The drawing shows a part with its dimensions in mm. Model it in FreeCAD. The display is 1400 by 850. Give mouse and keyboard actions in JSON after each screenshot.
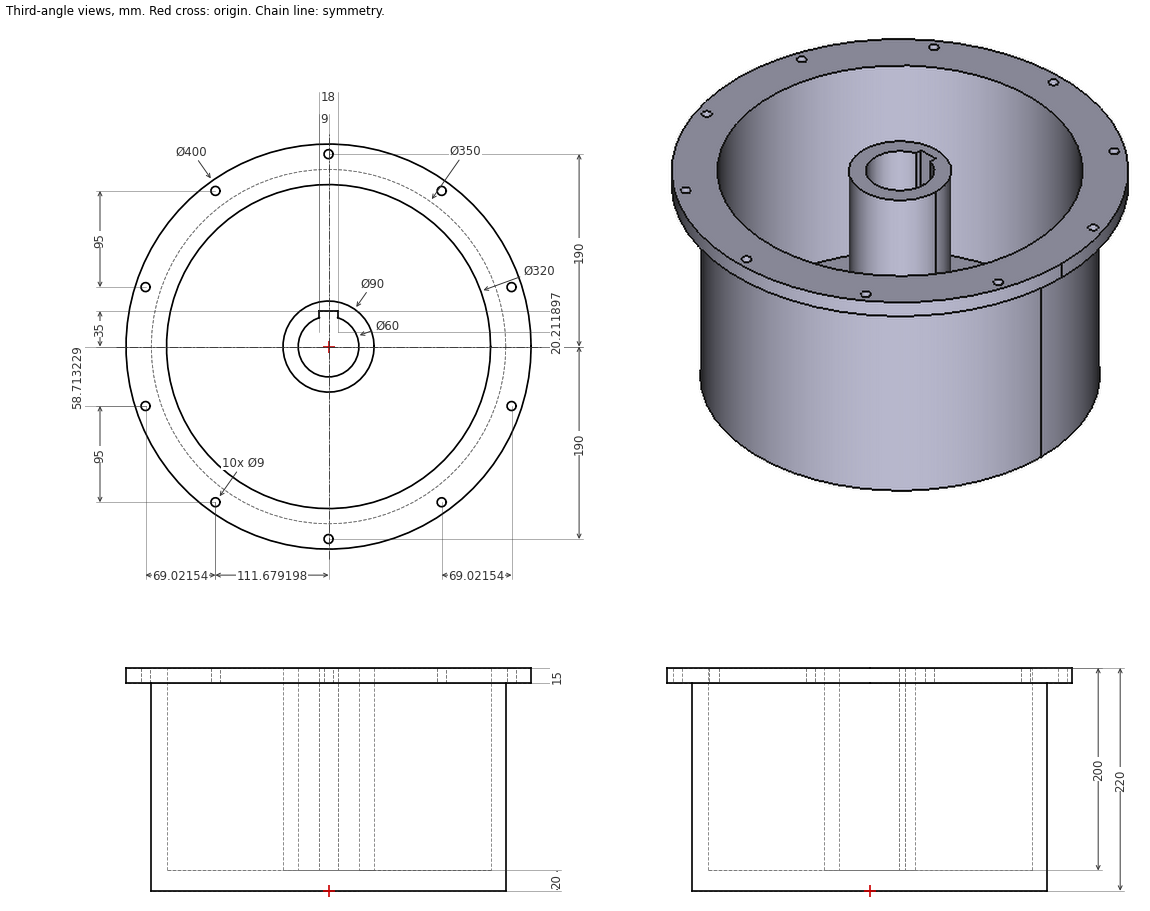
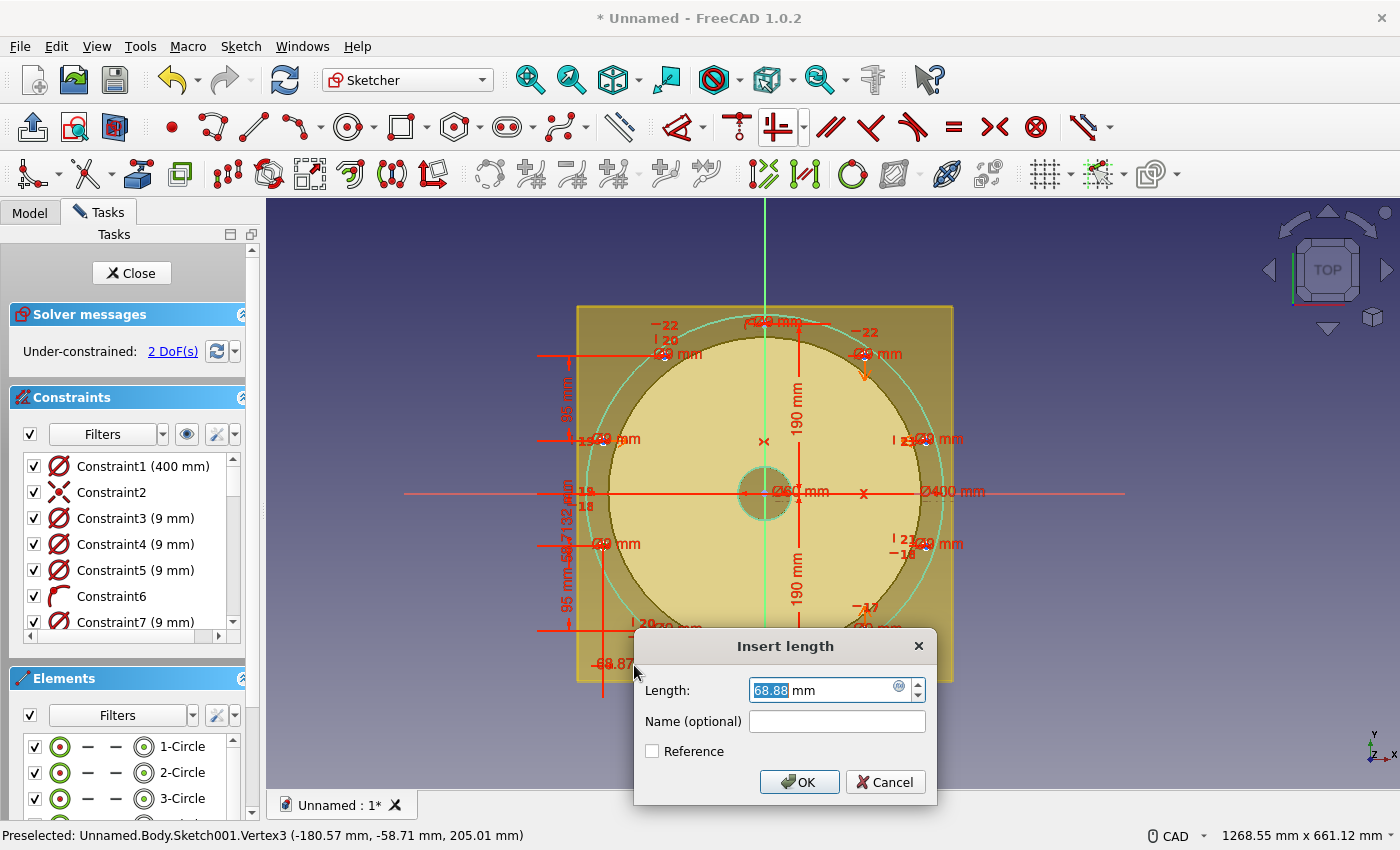
{"action": "type", "text": "69.02154"}
{"action": "key", "text": "Return"}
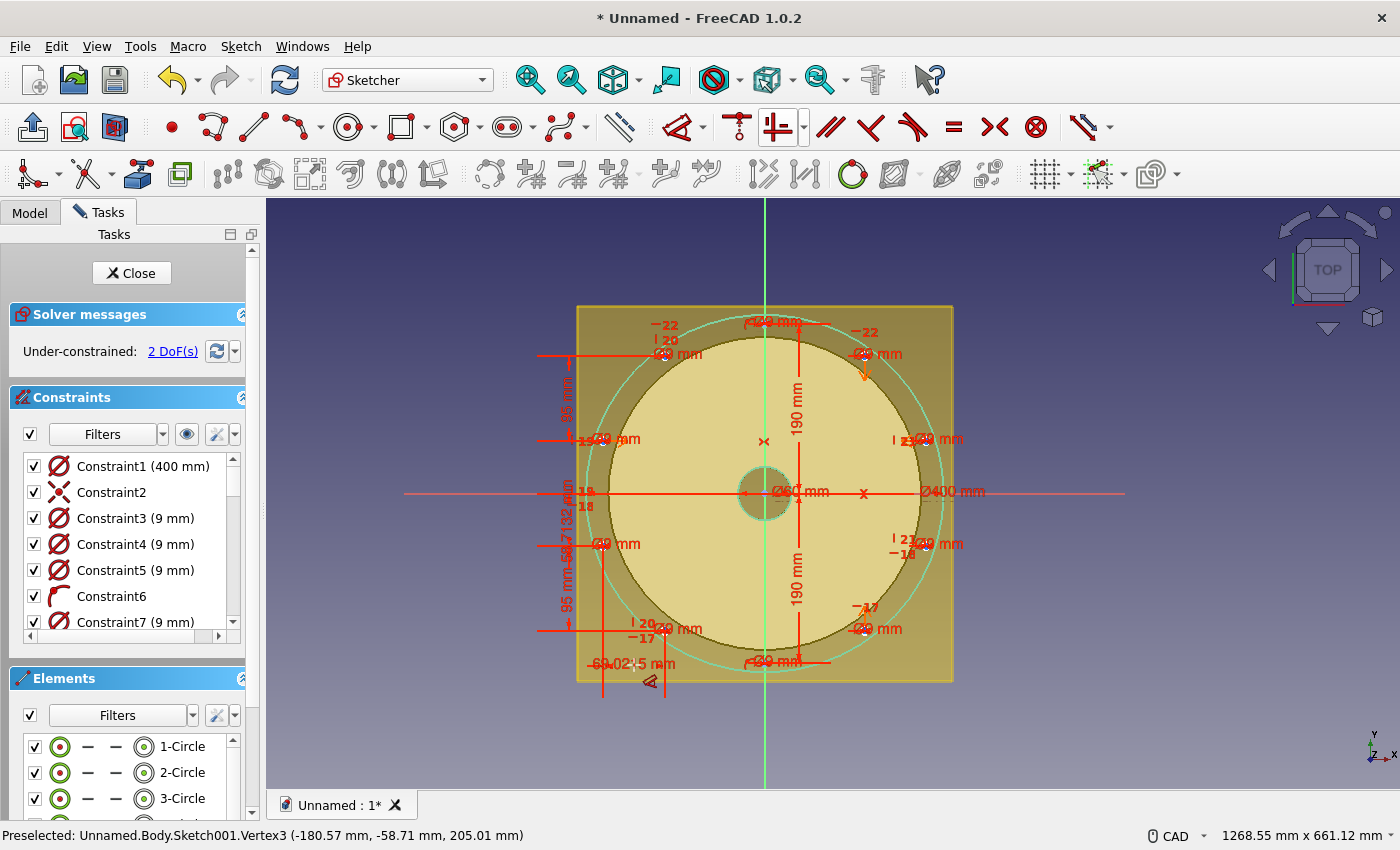
{"action": "left_click", "coordinate": [865, 631]}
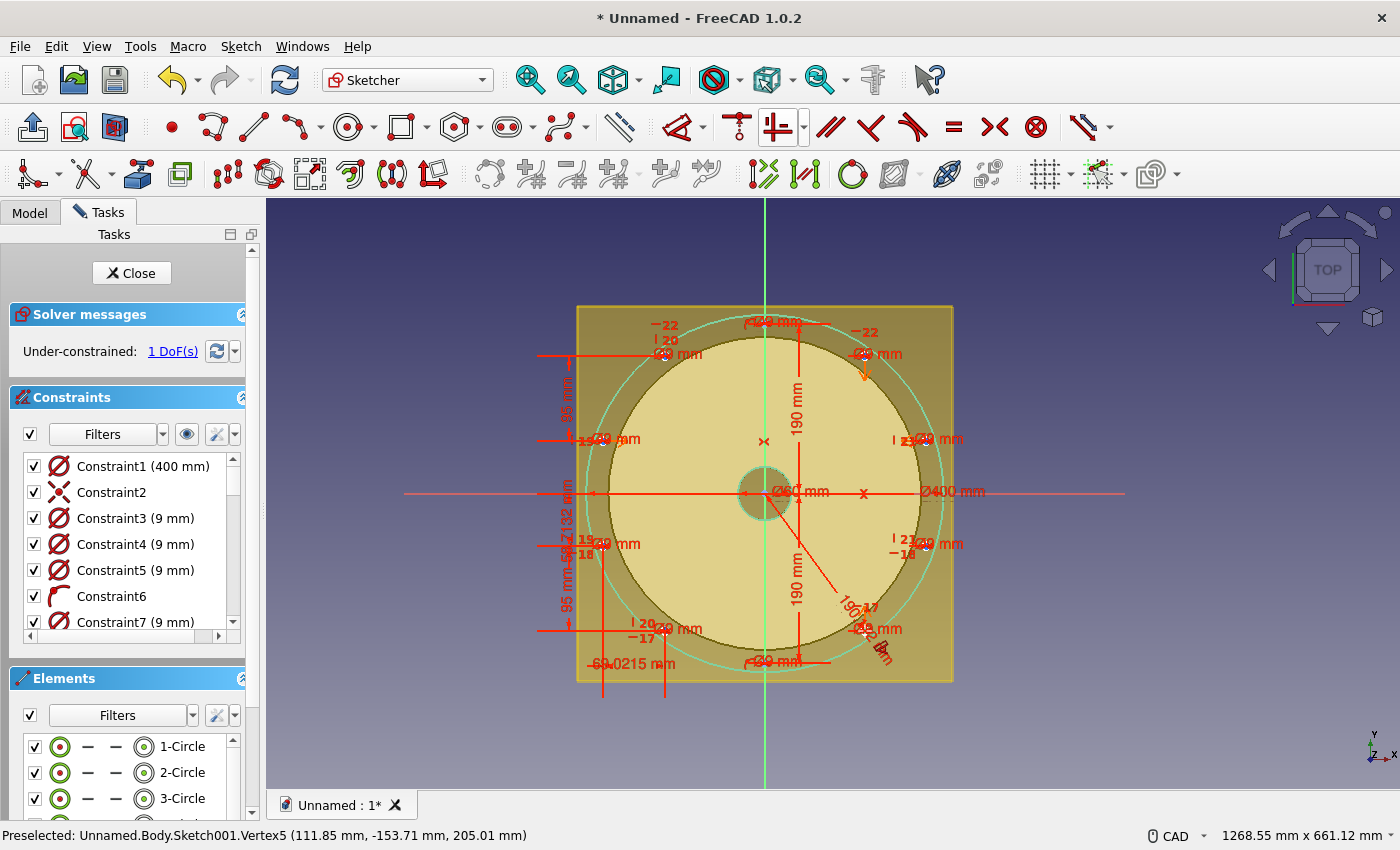
{"action": "left_click", "coordinate": [926, 546]}
{"action": "left_click", "coordinate": [896, 665]}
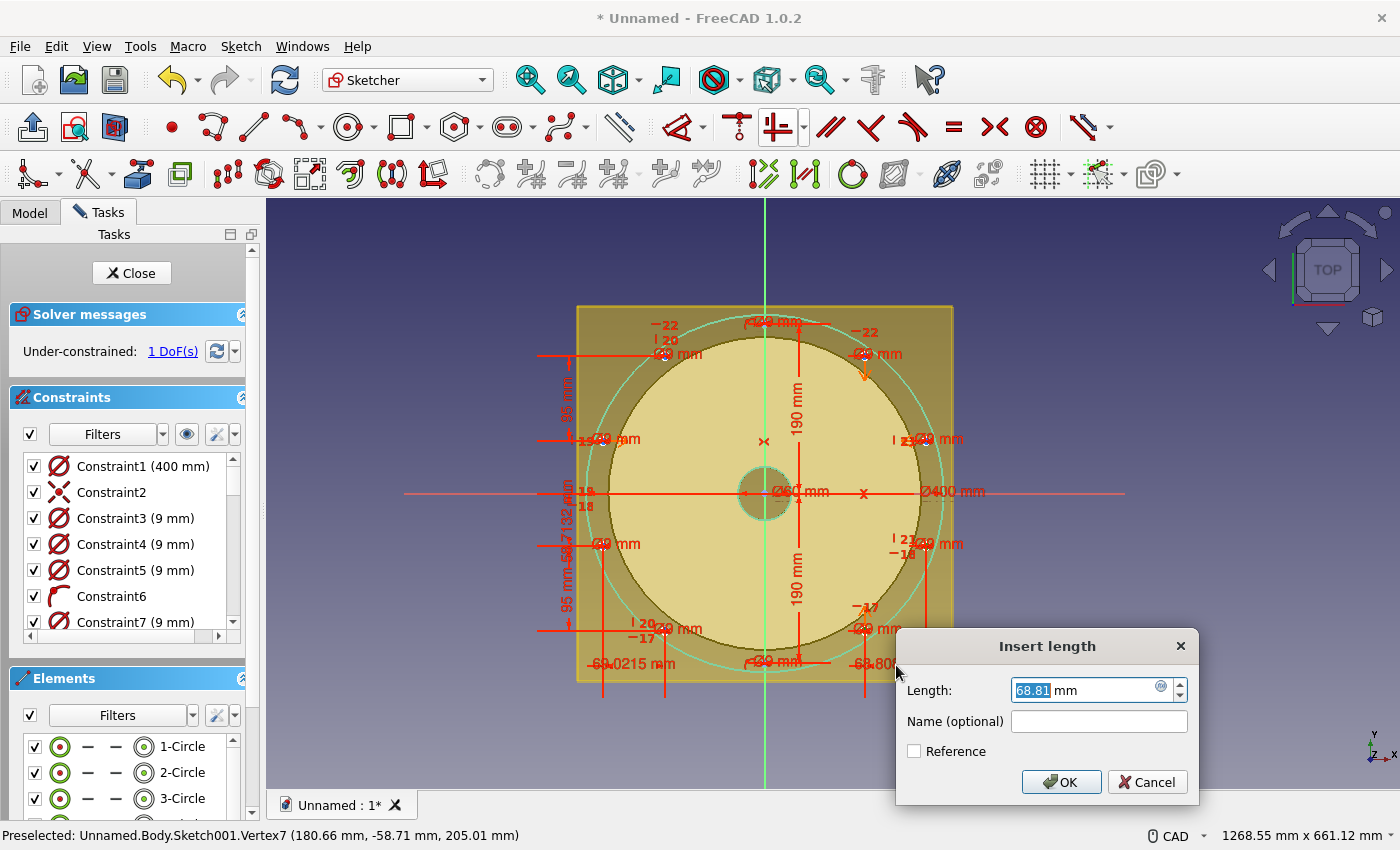
{"action": "type", "text": "69.02154"}
{"action": "key", "text": "Return"}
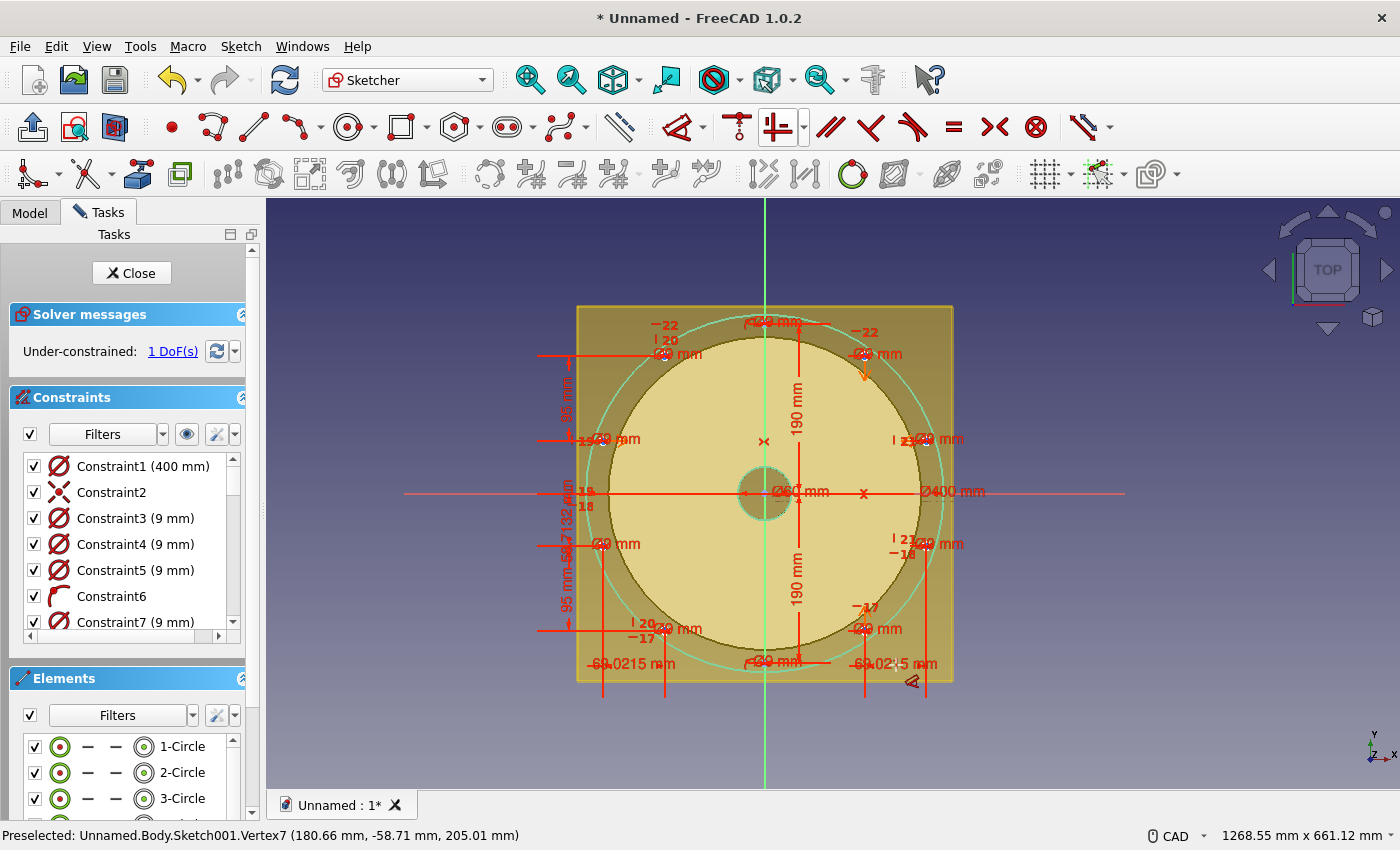
{"action": "left_click", "coordinate": [665, 631]}
{"action": "left_click", "coordinate": [715, 460]}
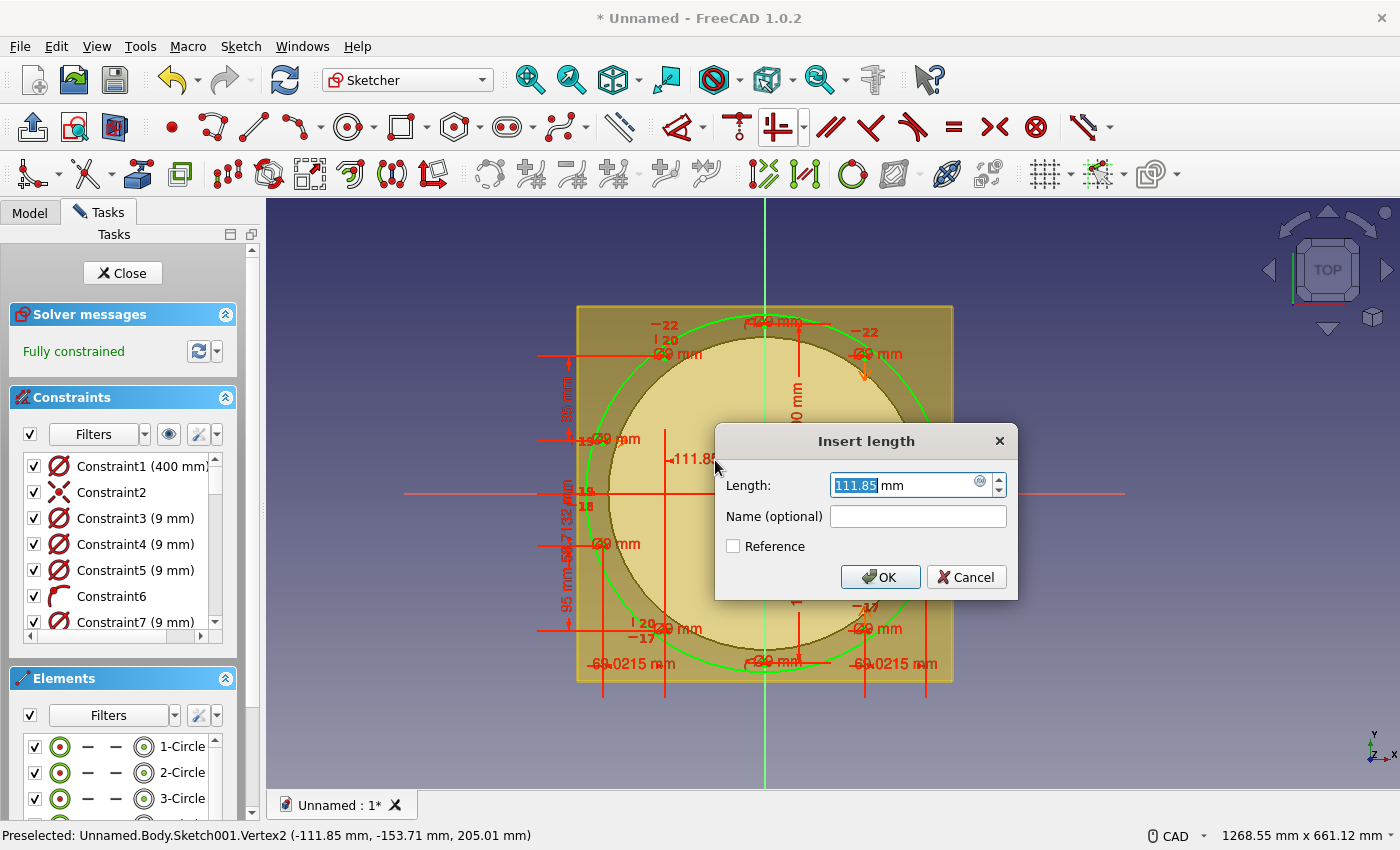
{"action": "type", "text": "111.679198"}
{"action": "key", "text": "Return"}
{"action": "key", "text": "Escape"}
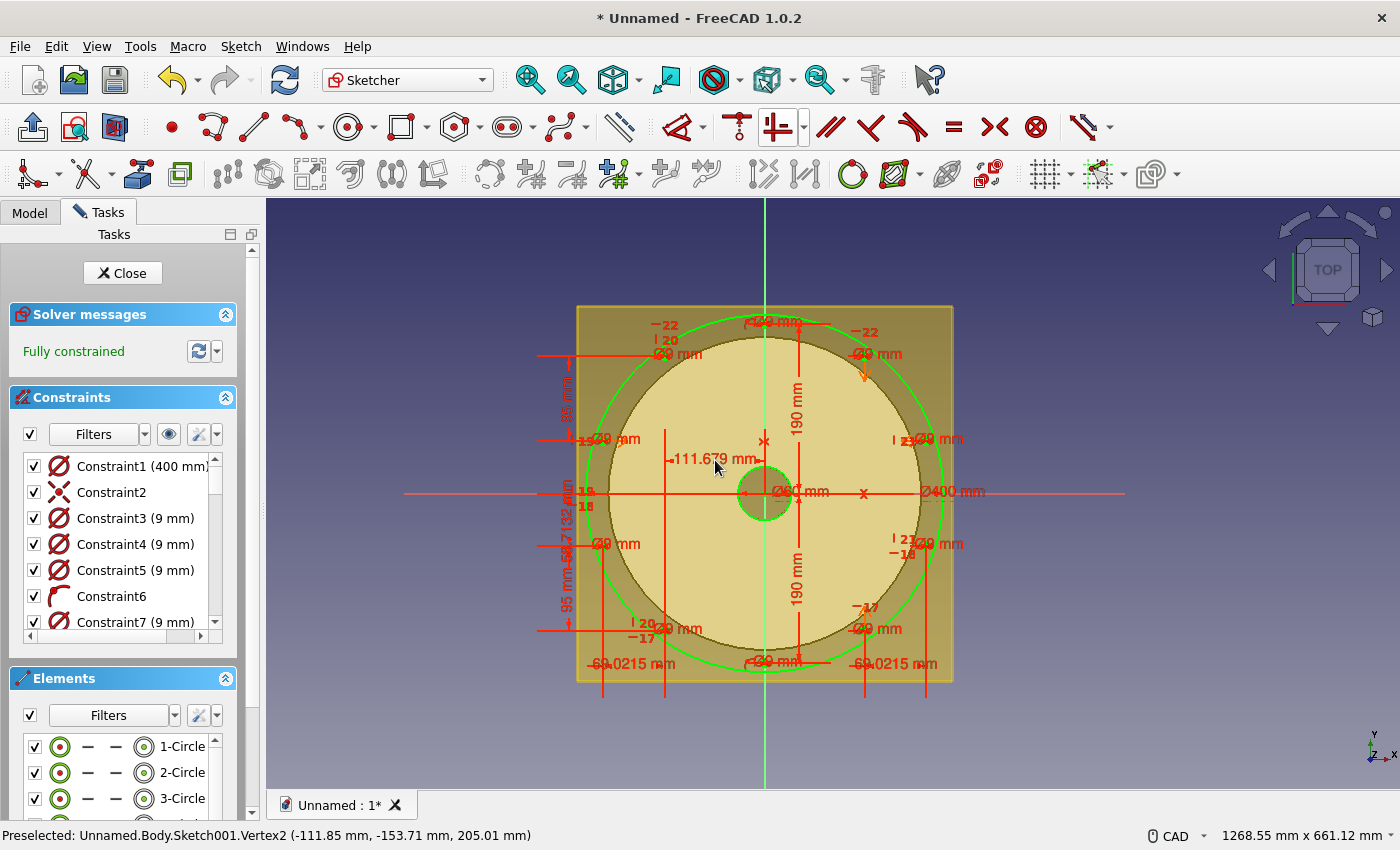
{"action": "left_click", "coordinate": [123, 273]}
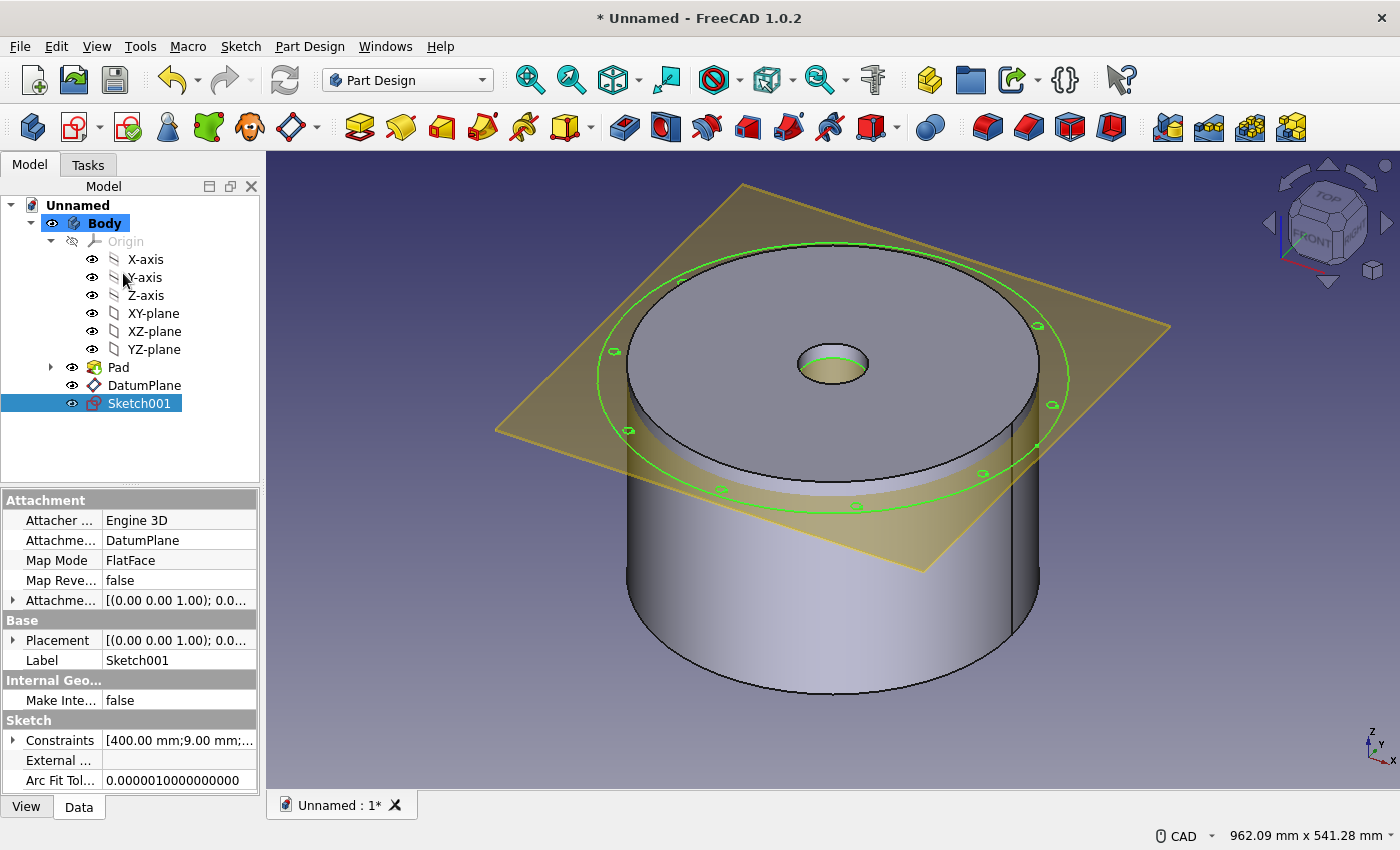
{"action": "left_click", "coordinate": [360, 128]}